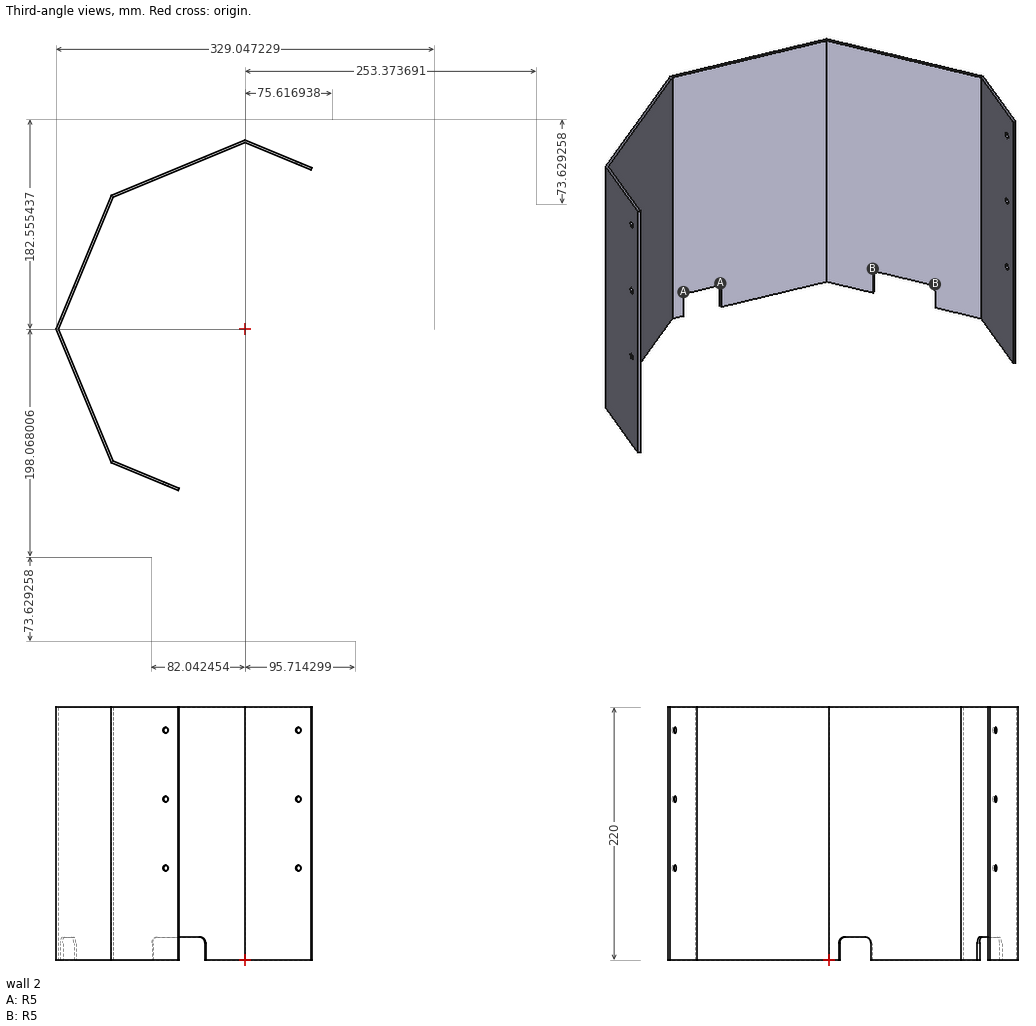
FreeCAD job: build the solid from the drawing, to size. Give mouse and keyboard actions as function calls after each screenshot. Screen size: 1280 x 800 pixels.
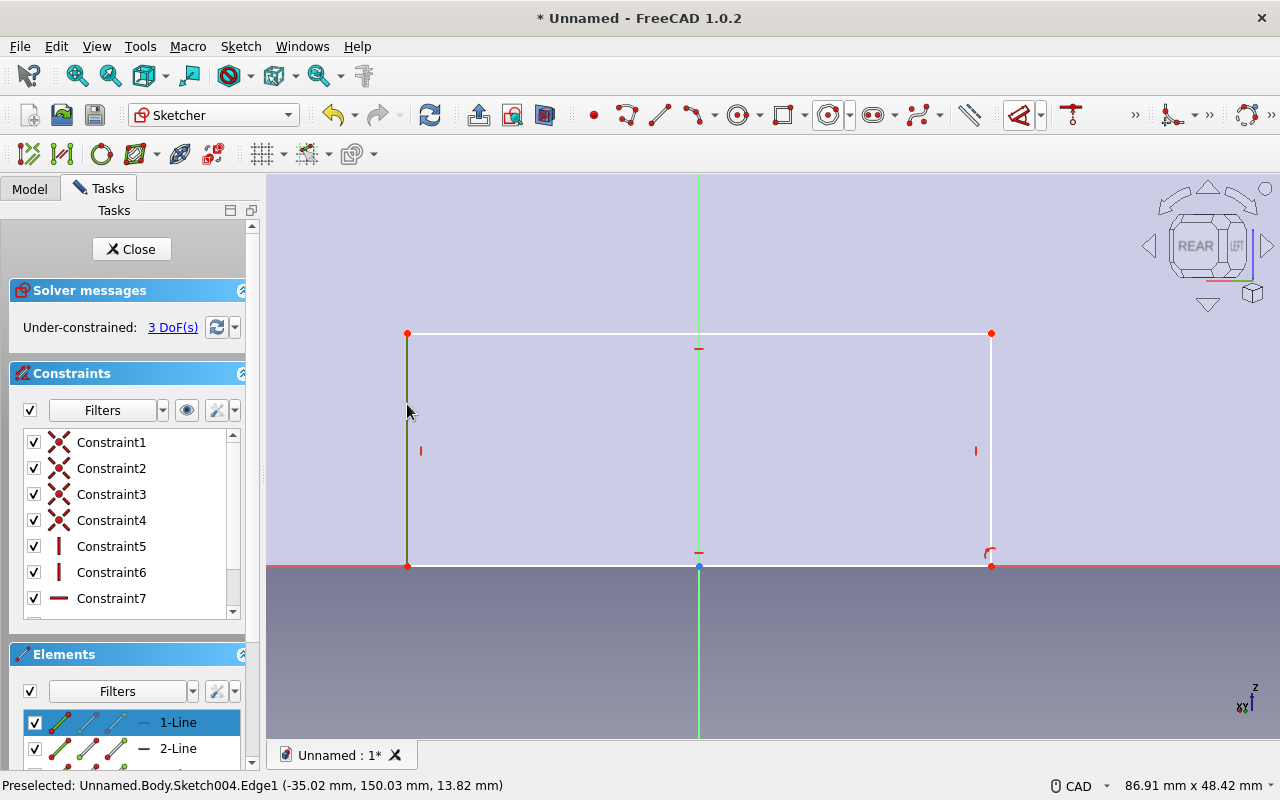
click(1040, 116)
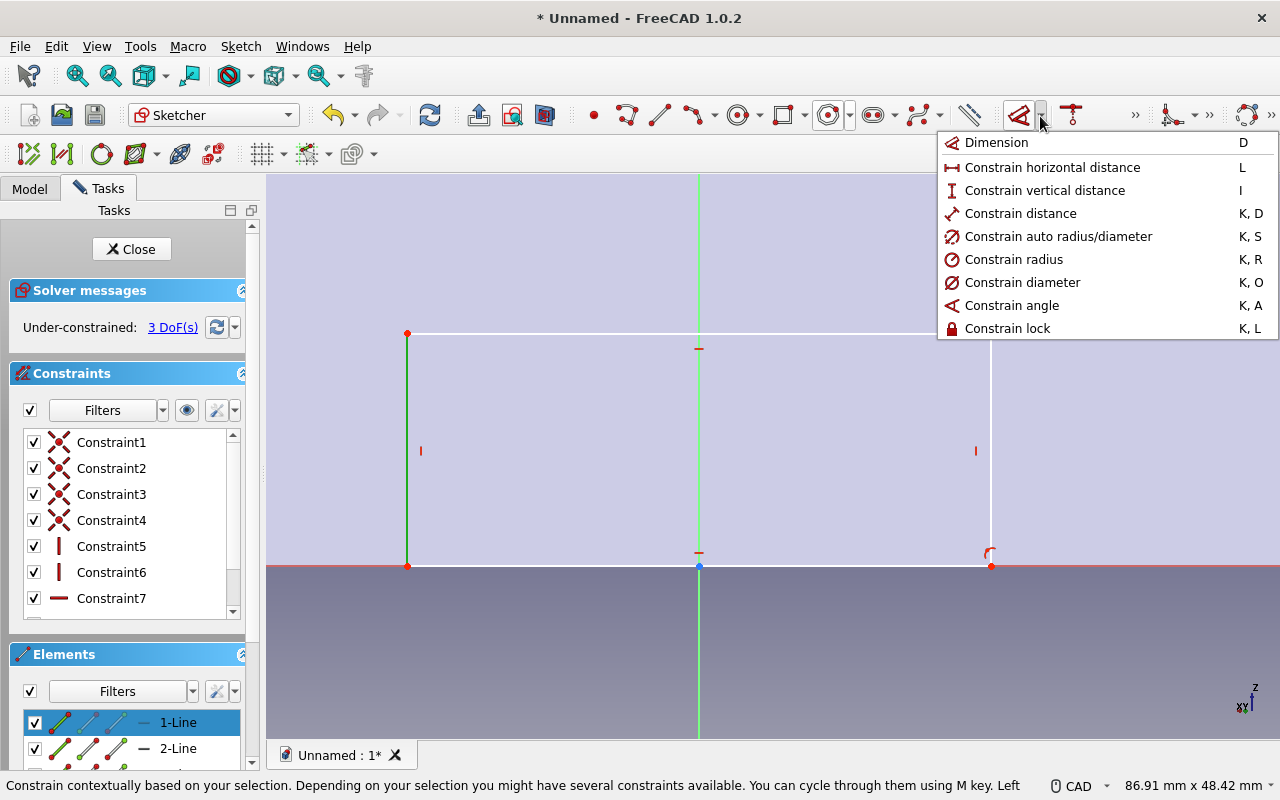
click(1108, 190)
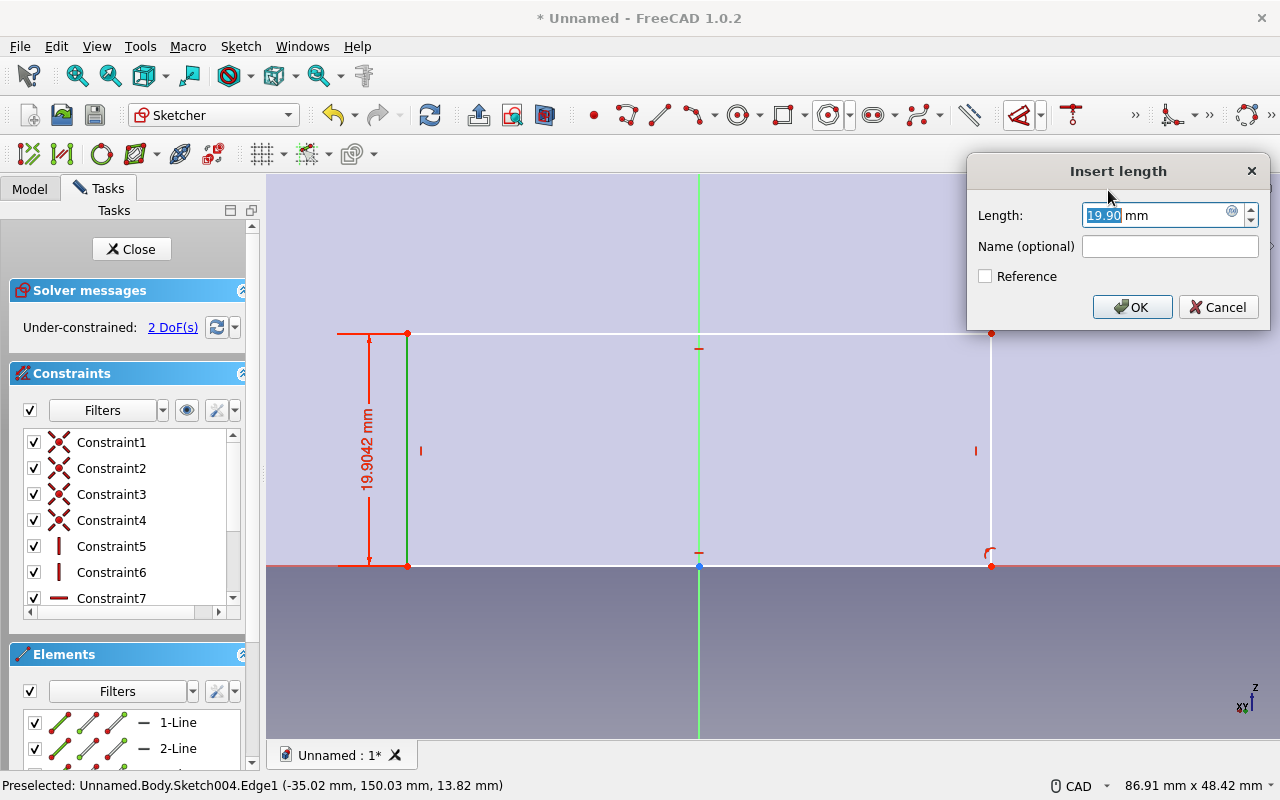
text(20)
key(Return)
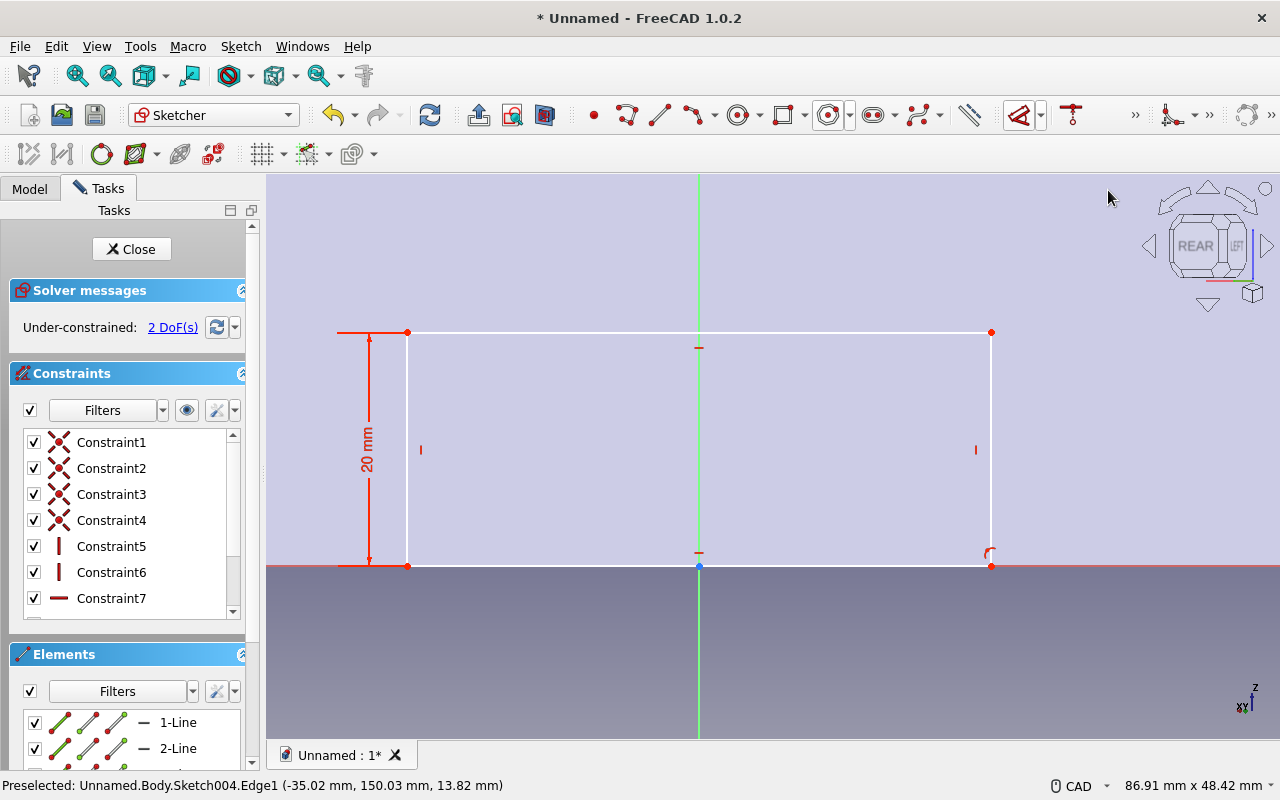
click(582, 566)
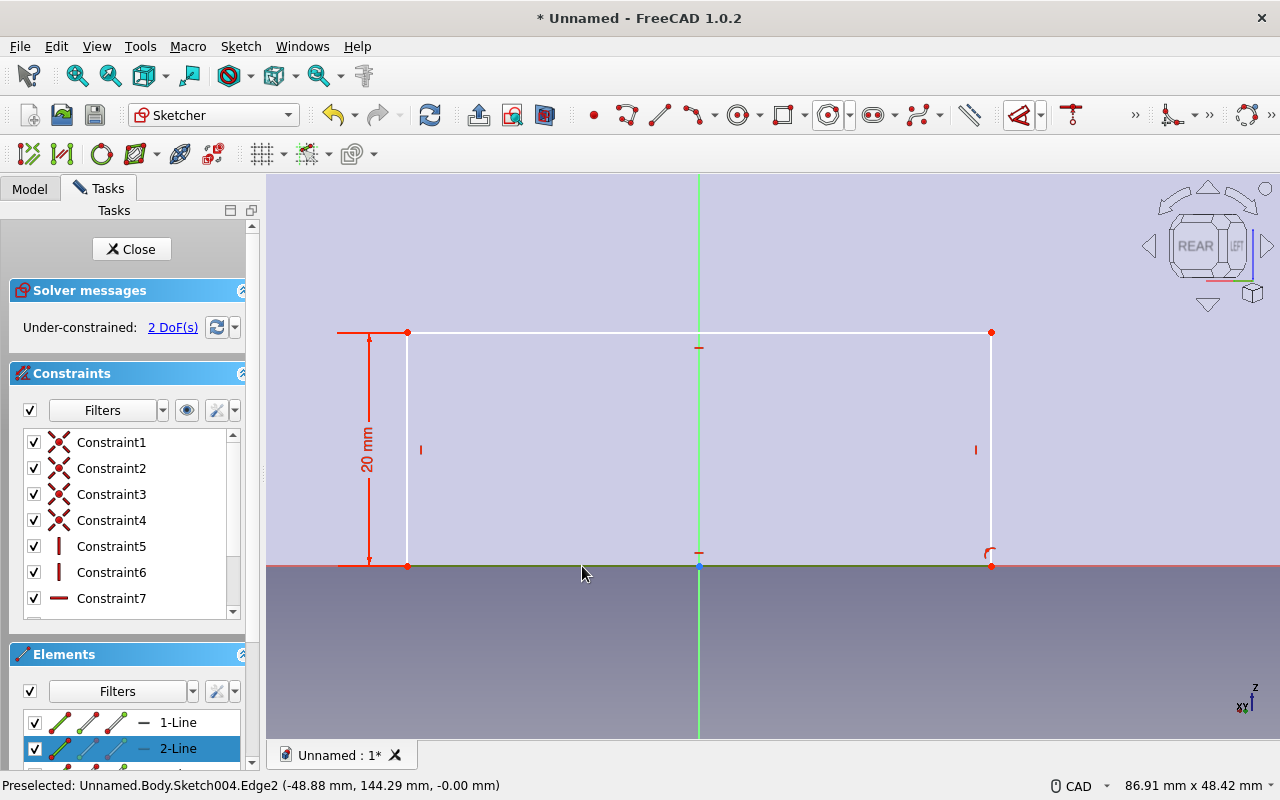
click(1040, 116)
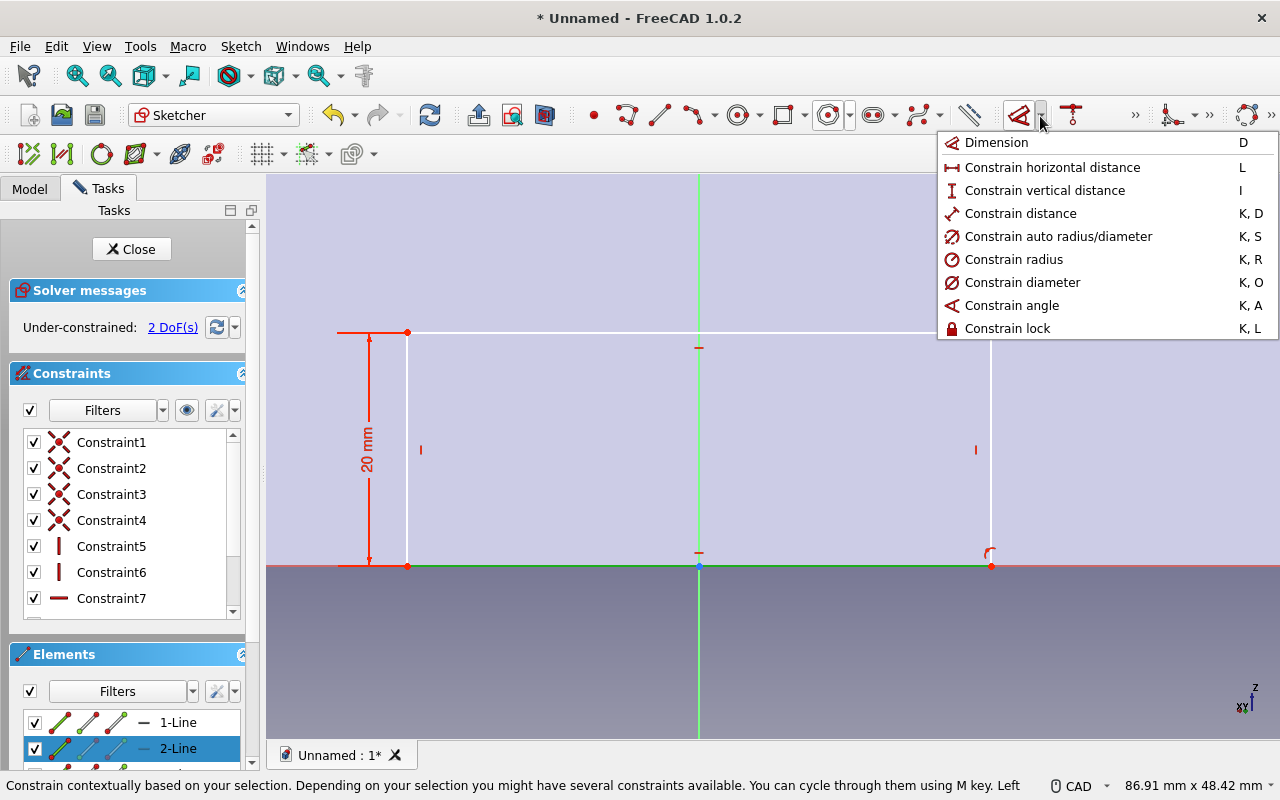
click(1108, 168)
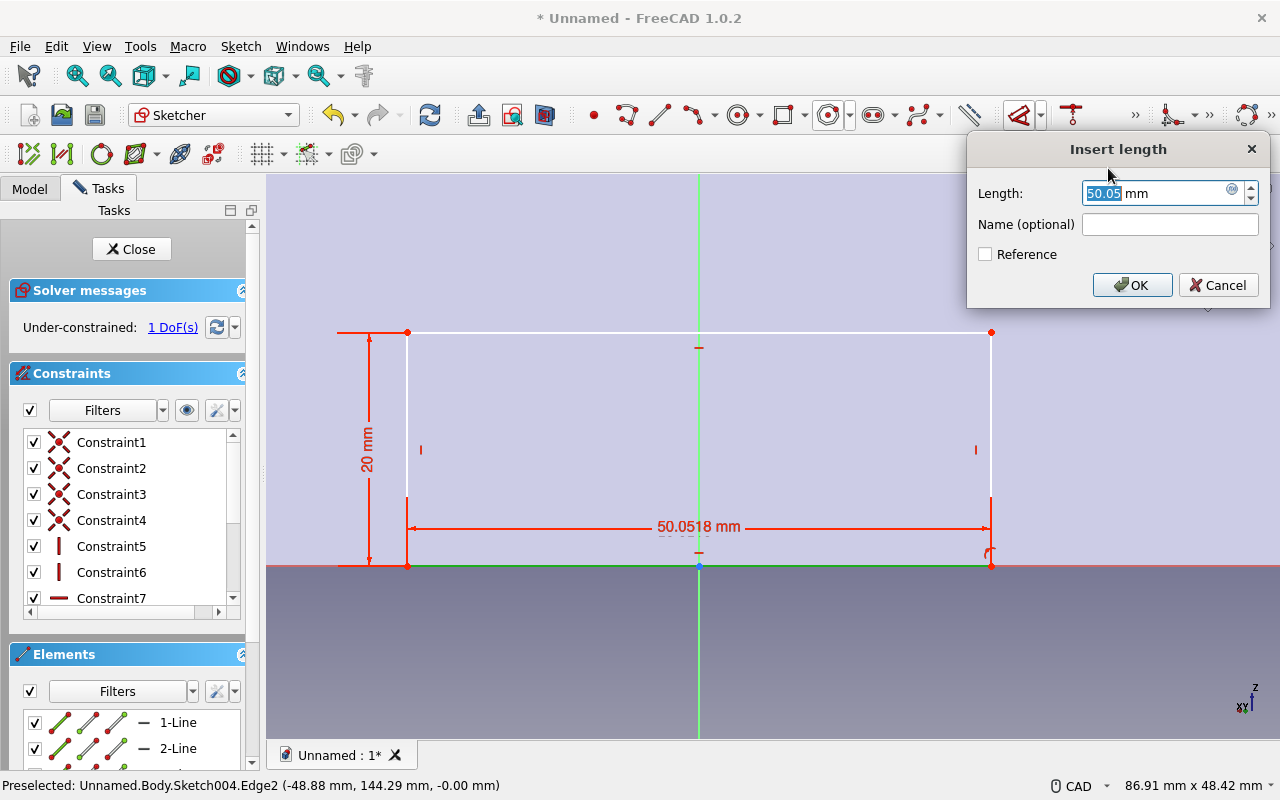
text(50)
key(Return)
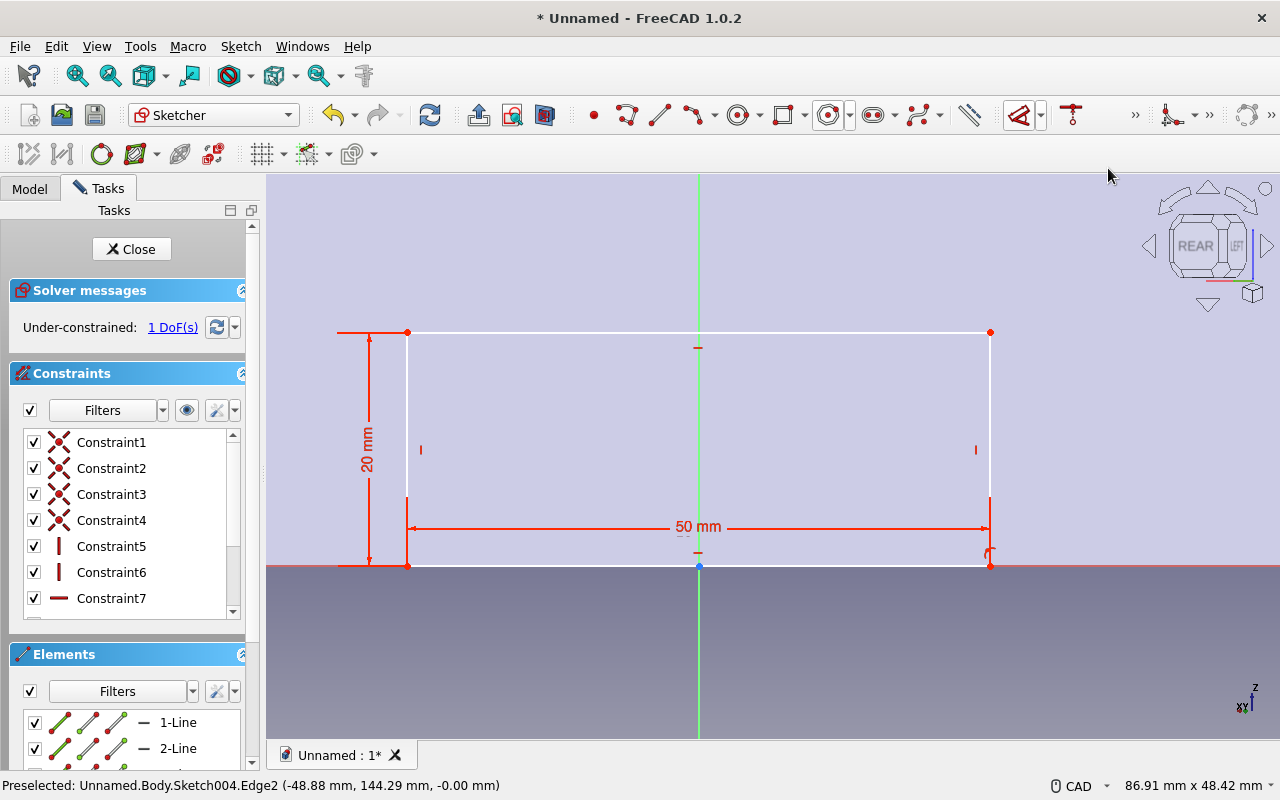
click(407, 333)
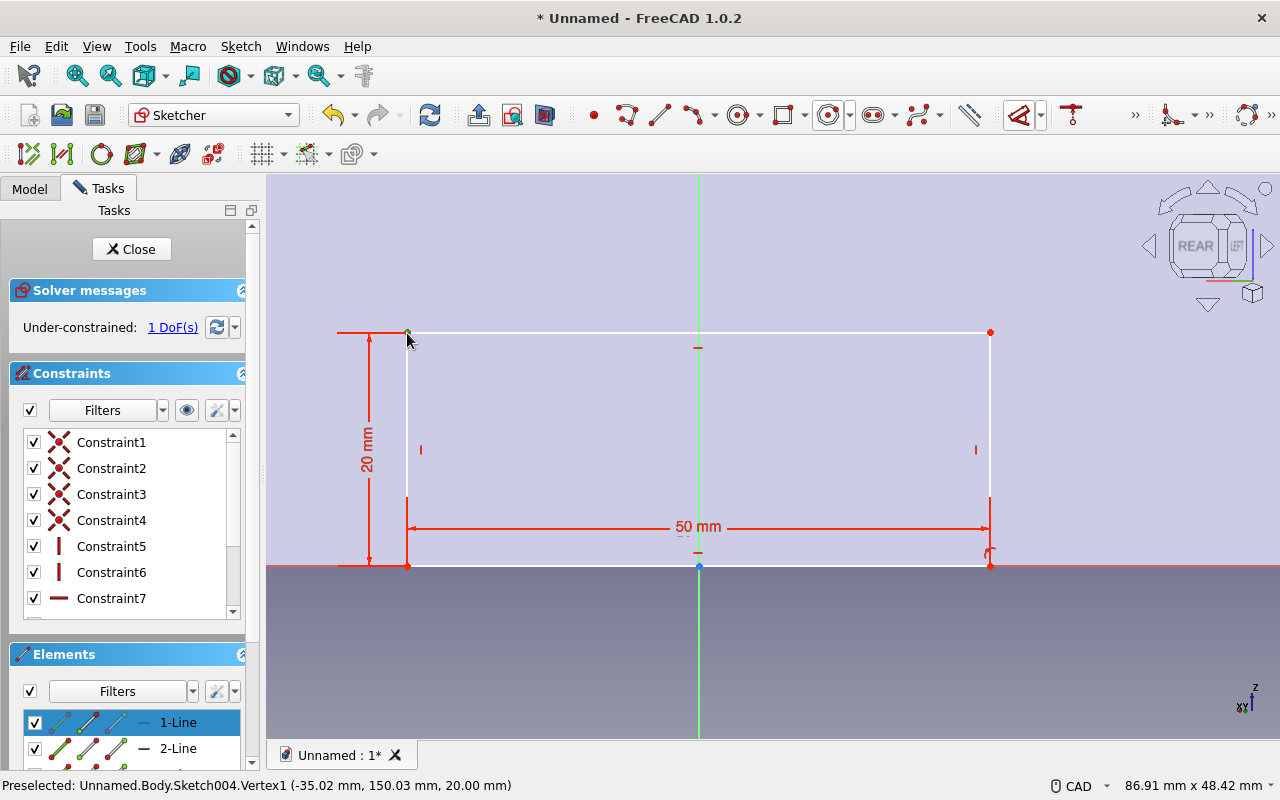
click(1040, 116)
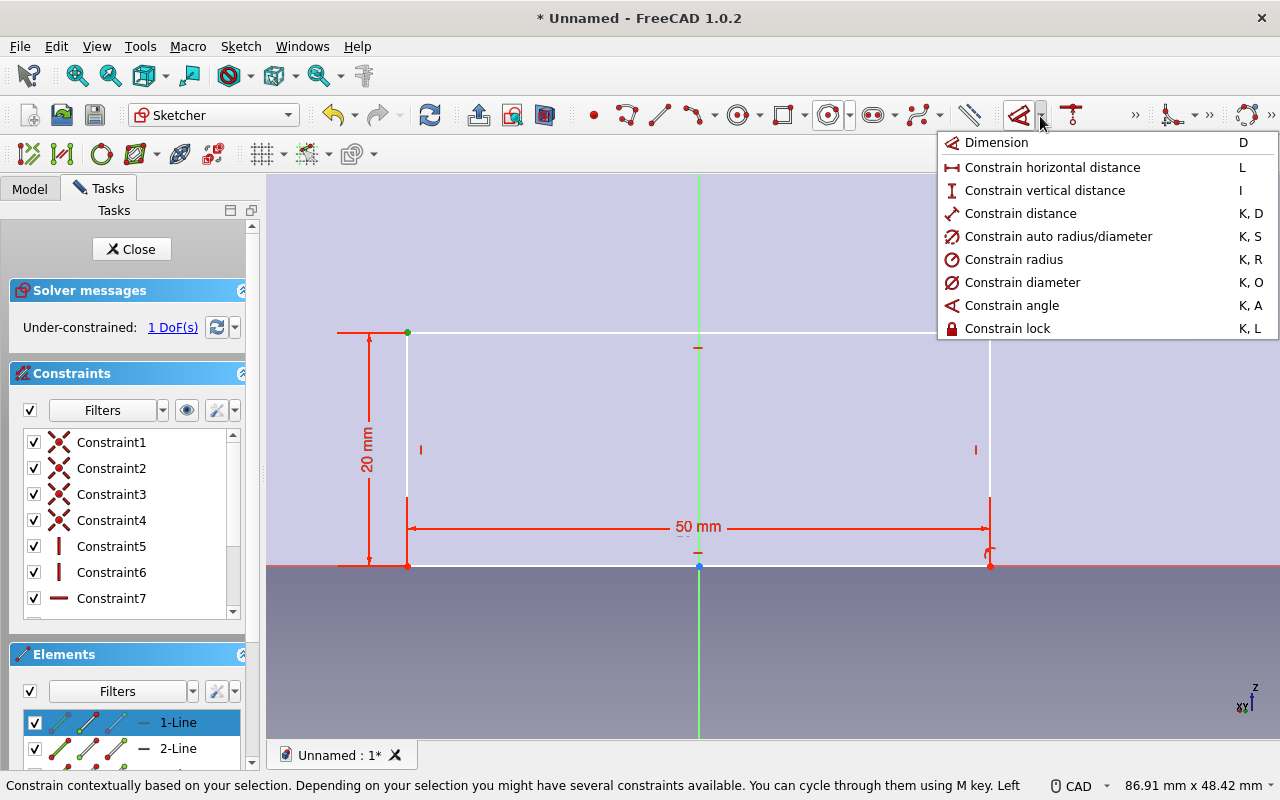
click(1108, 168)